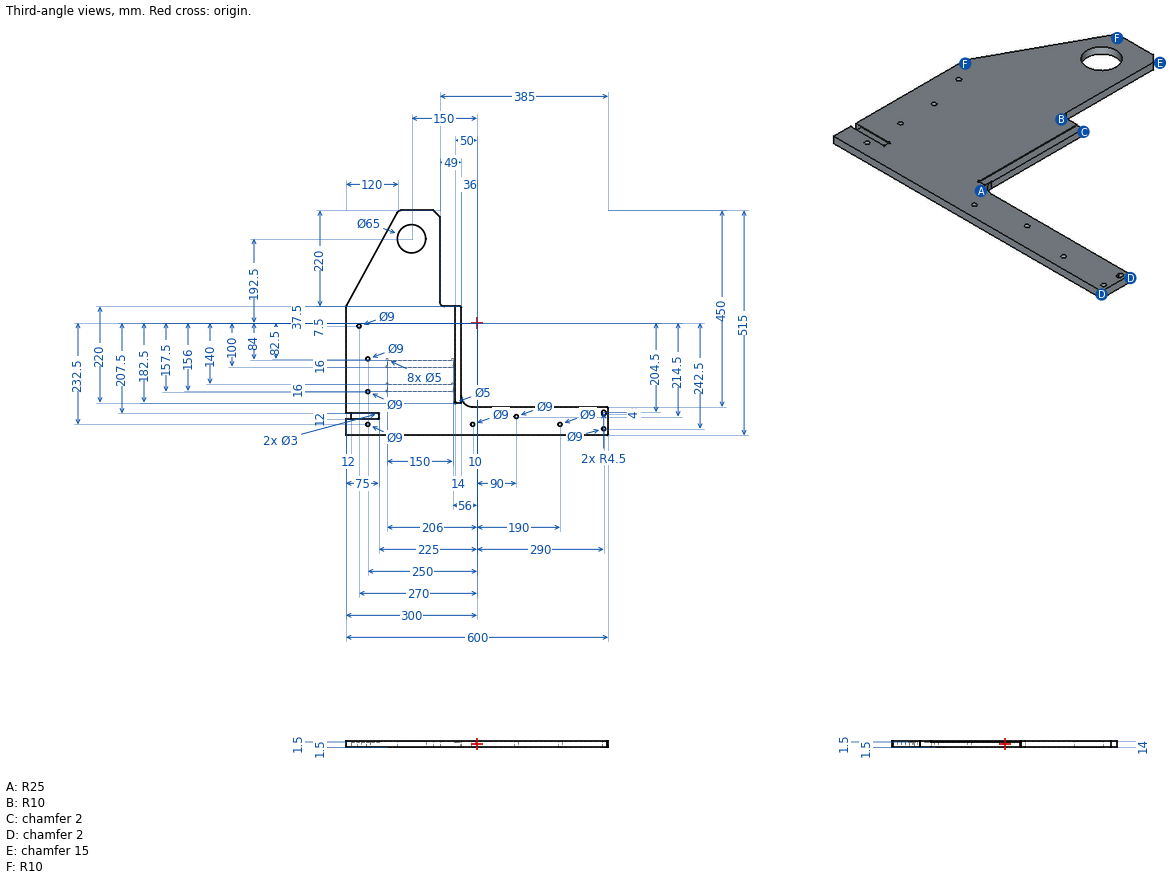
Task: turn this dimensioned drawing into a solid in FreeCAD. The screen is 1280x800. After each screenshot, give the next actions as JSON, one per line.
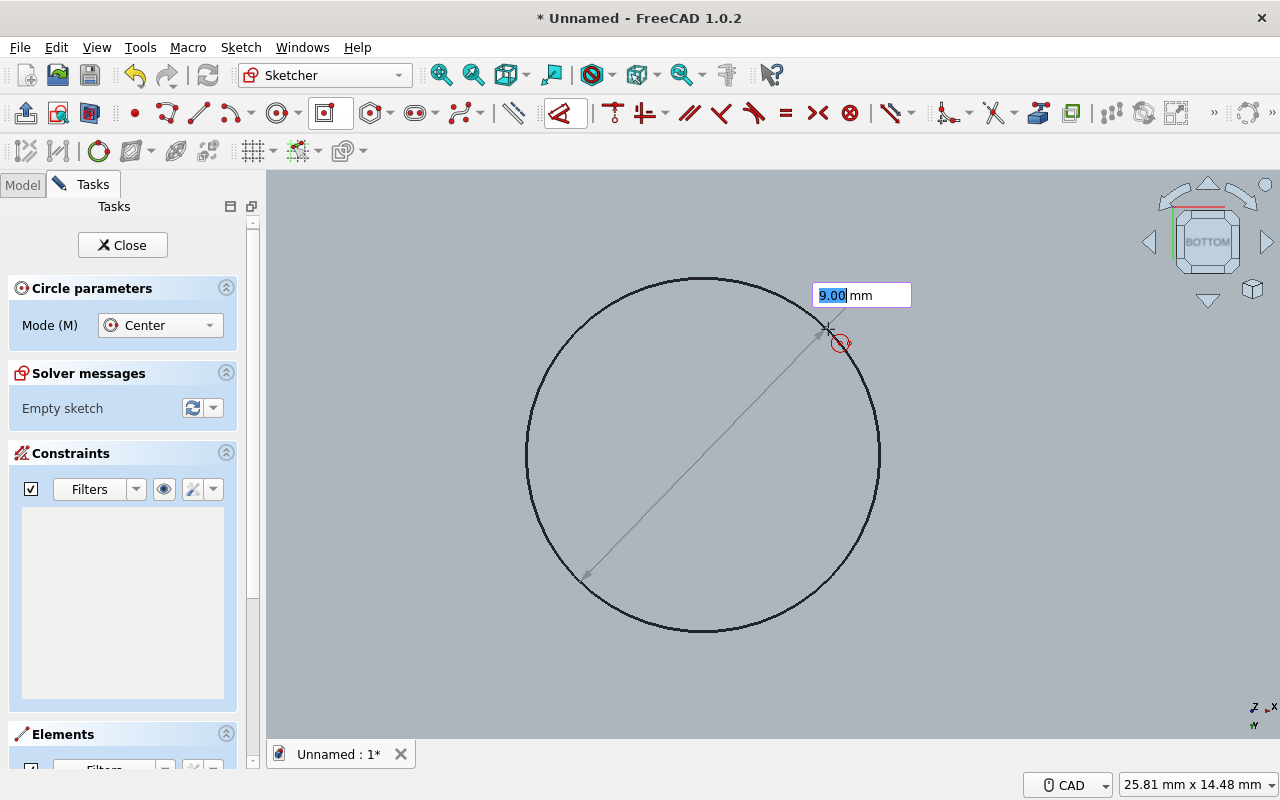
{"action": "type", "text": "9"}
{"action": "key", "text": "Return"}
{"action": "key", "text": "Escape"}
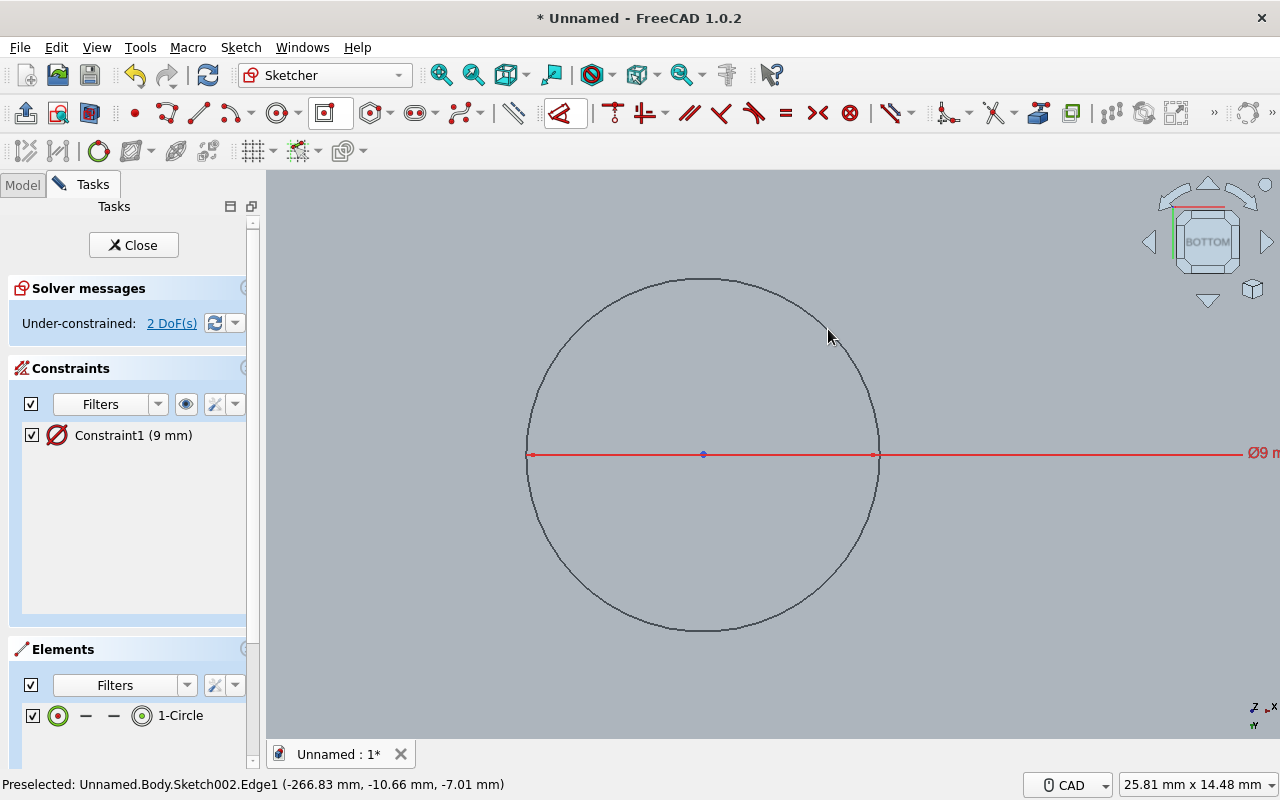
{"action": "left_click", "coordinate": [703, 455]}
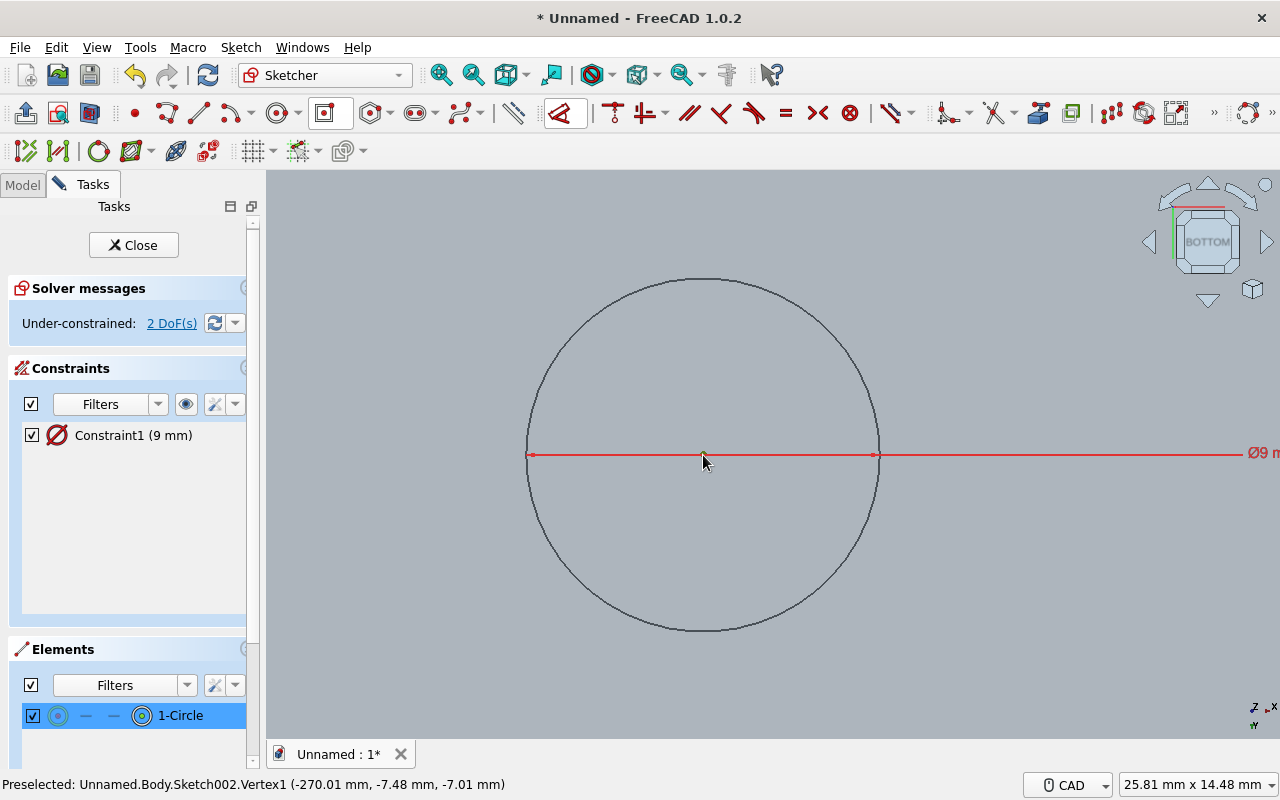
{"action": "left_click", "coordinate": [582, 114]}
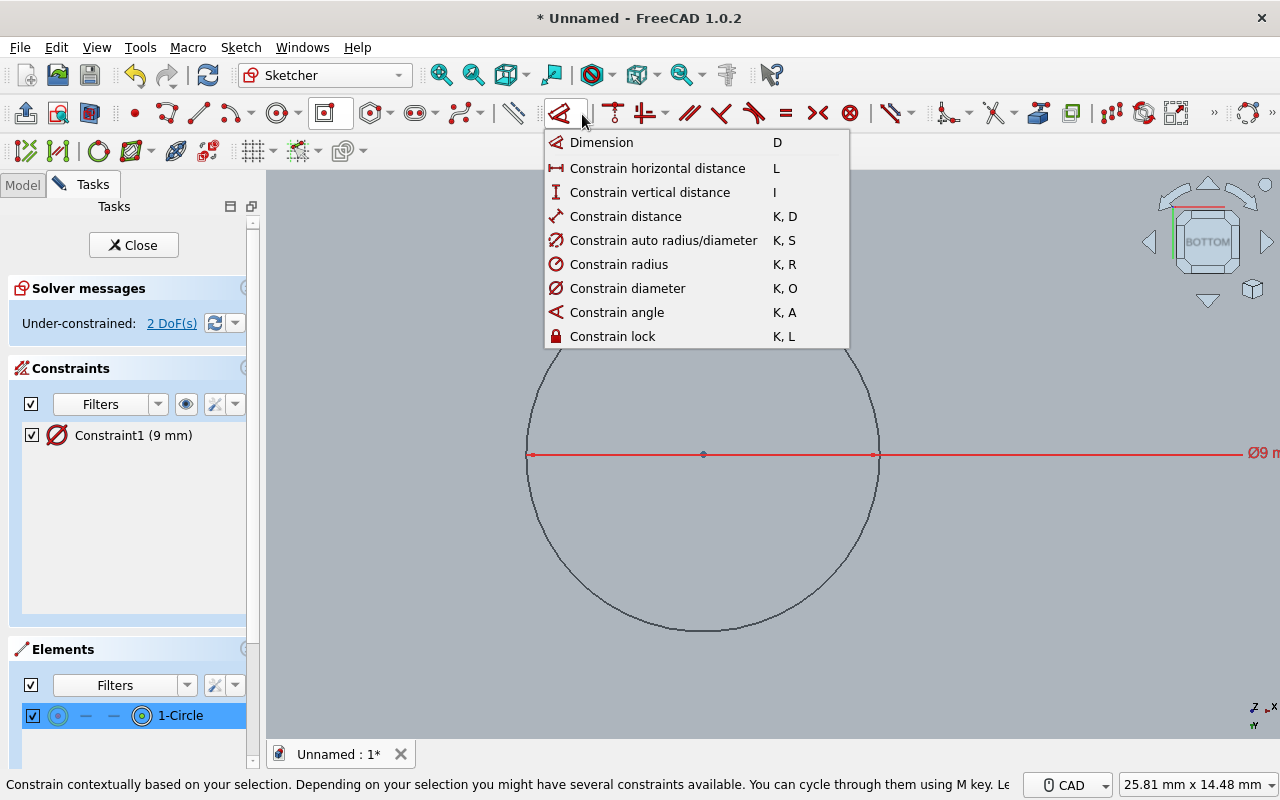
{"action": "left_click", "coordinate": [697, 168]}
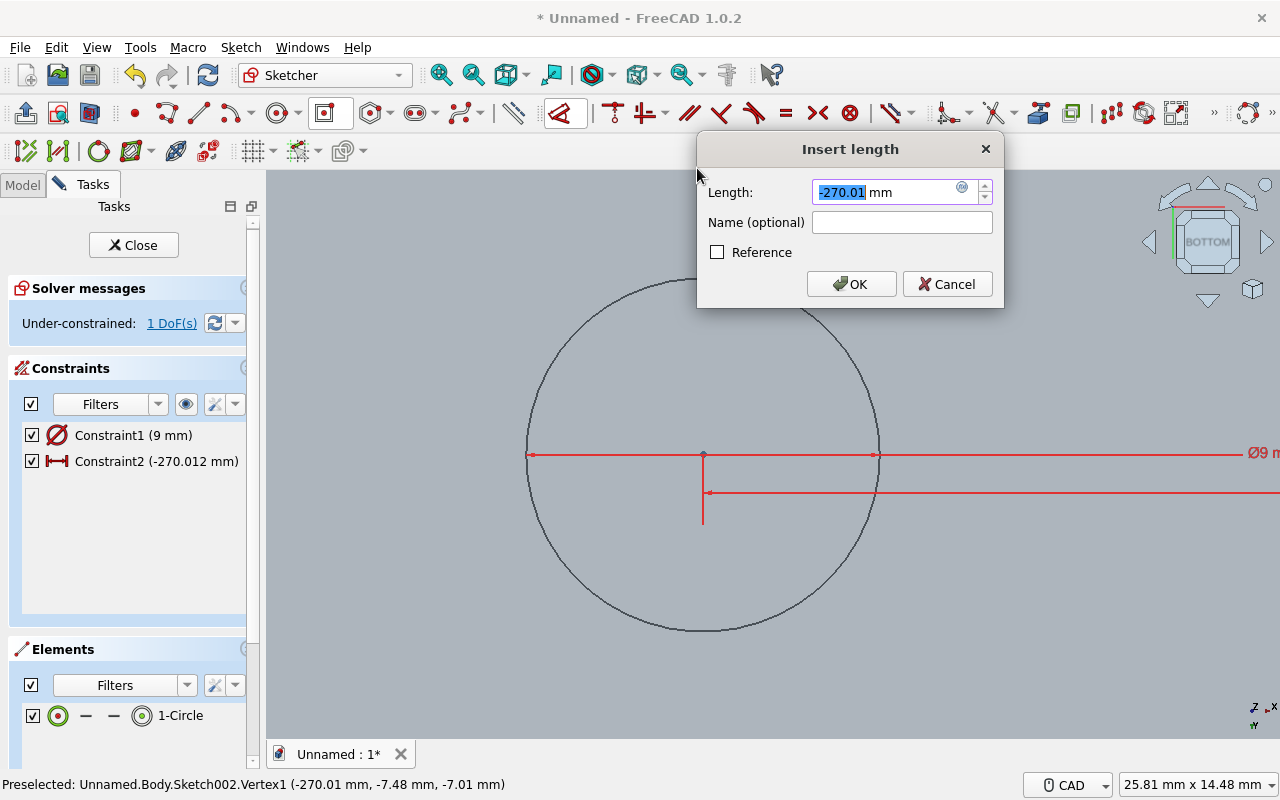
{"action": "type", "text": "-270"}
{"action": "key", "text": "Return"}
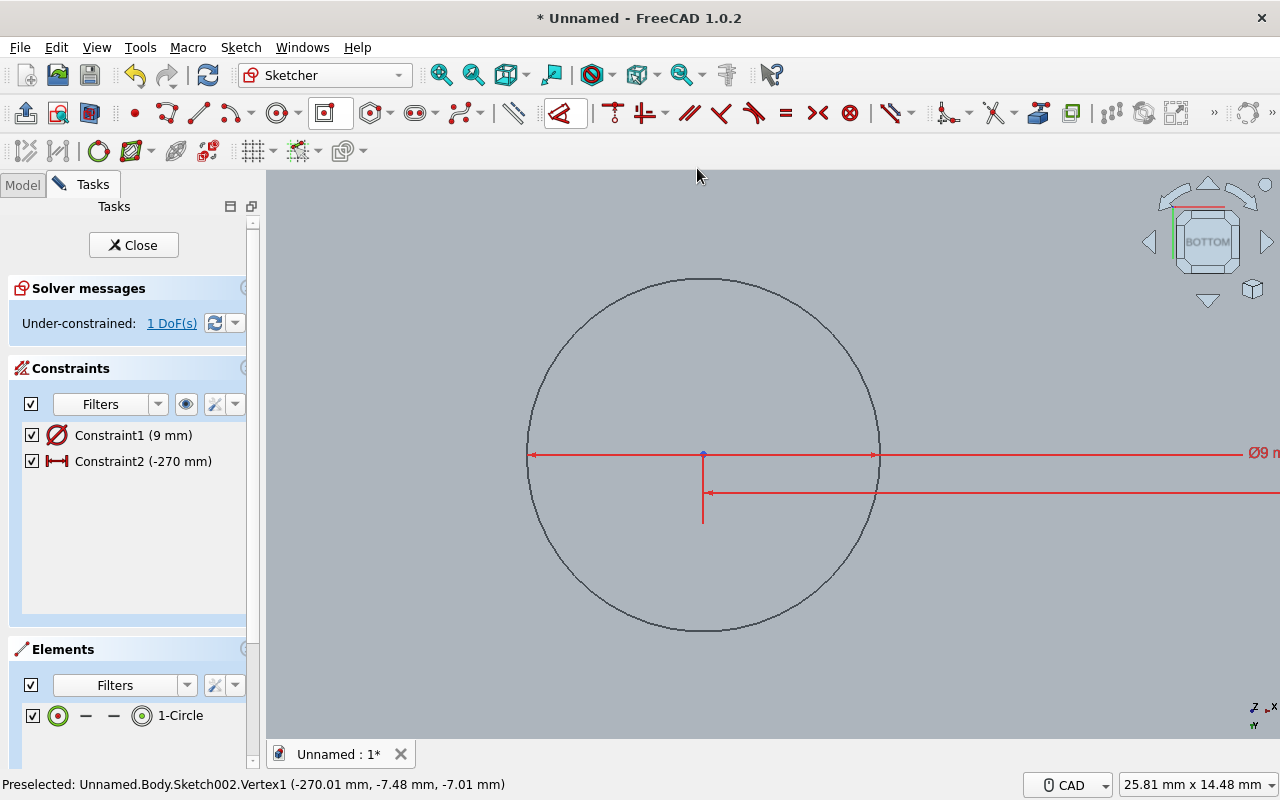
{"action": "left_click", "coordinate": [703, 455]}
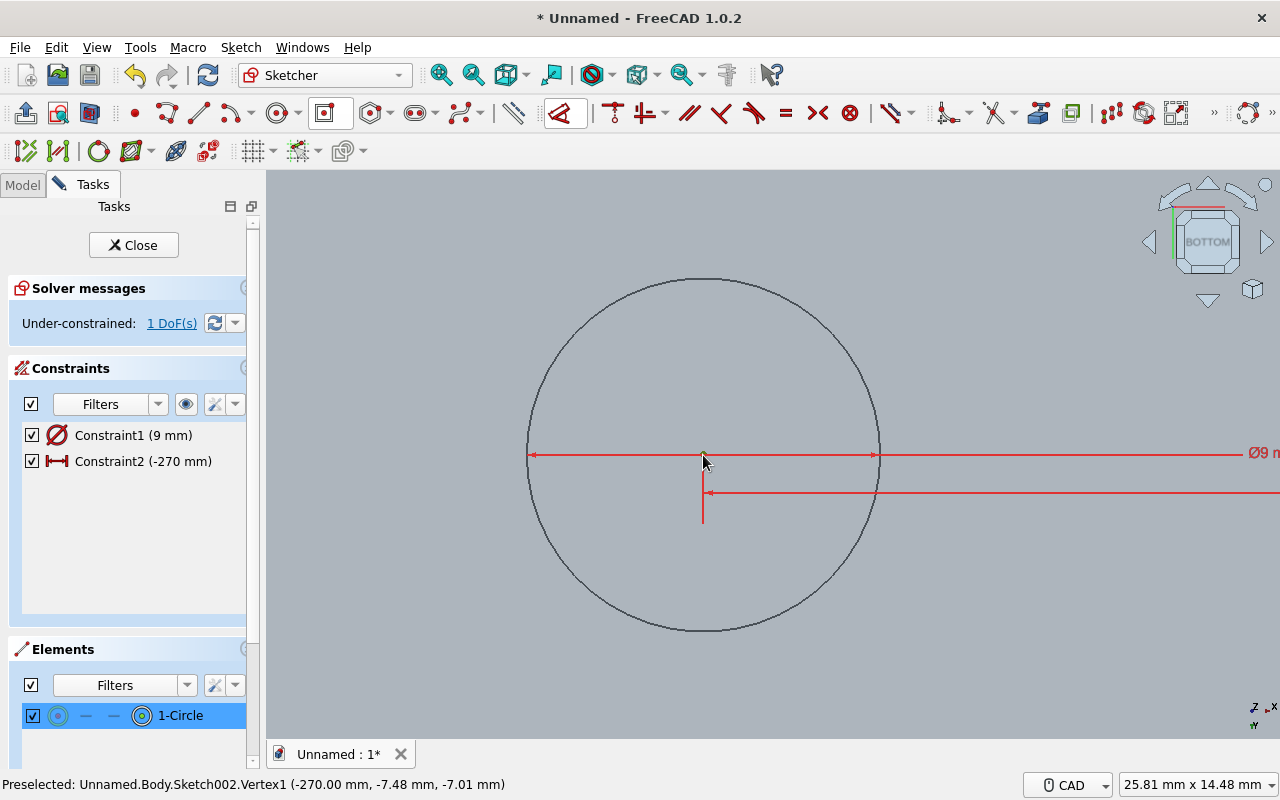
{"action": "key", "text": "i"}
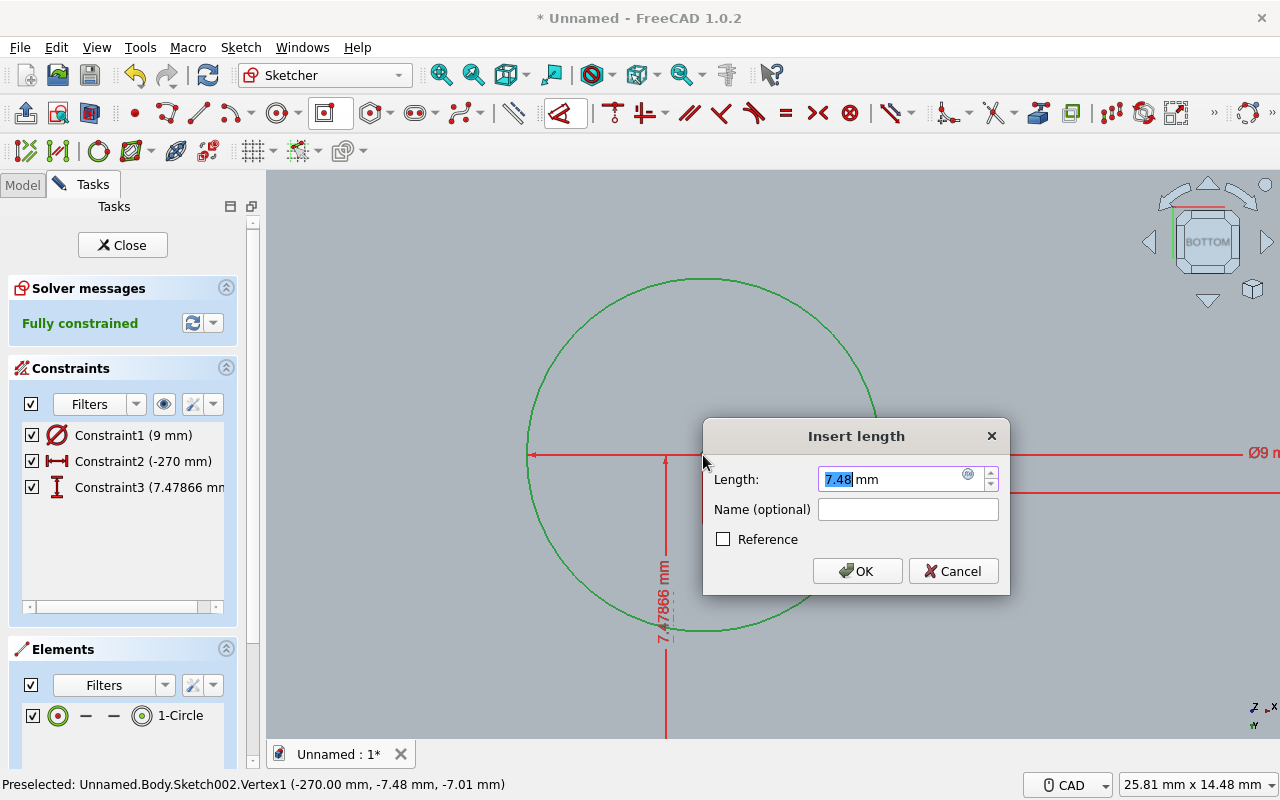
{"action": "type", "text": "7.5"}
{"action": "key", "text": "Return"}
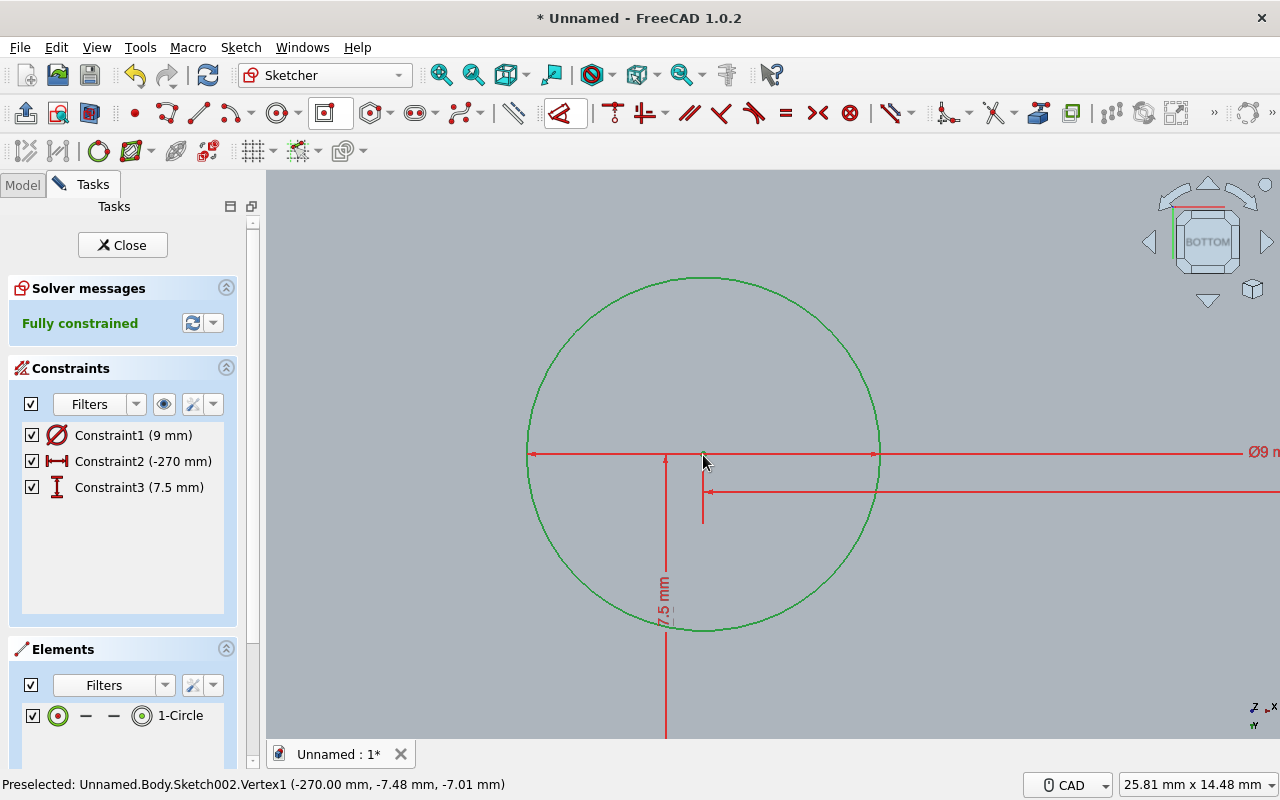
{"action": "left_click", "coordinate": [123, 245]}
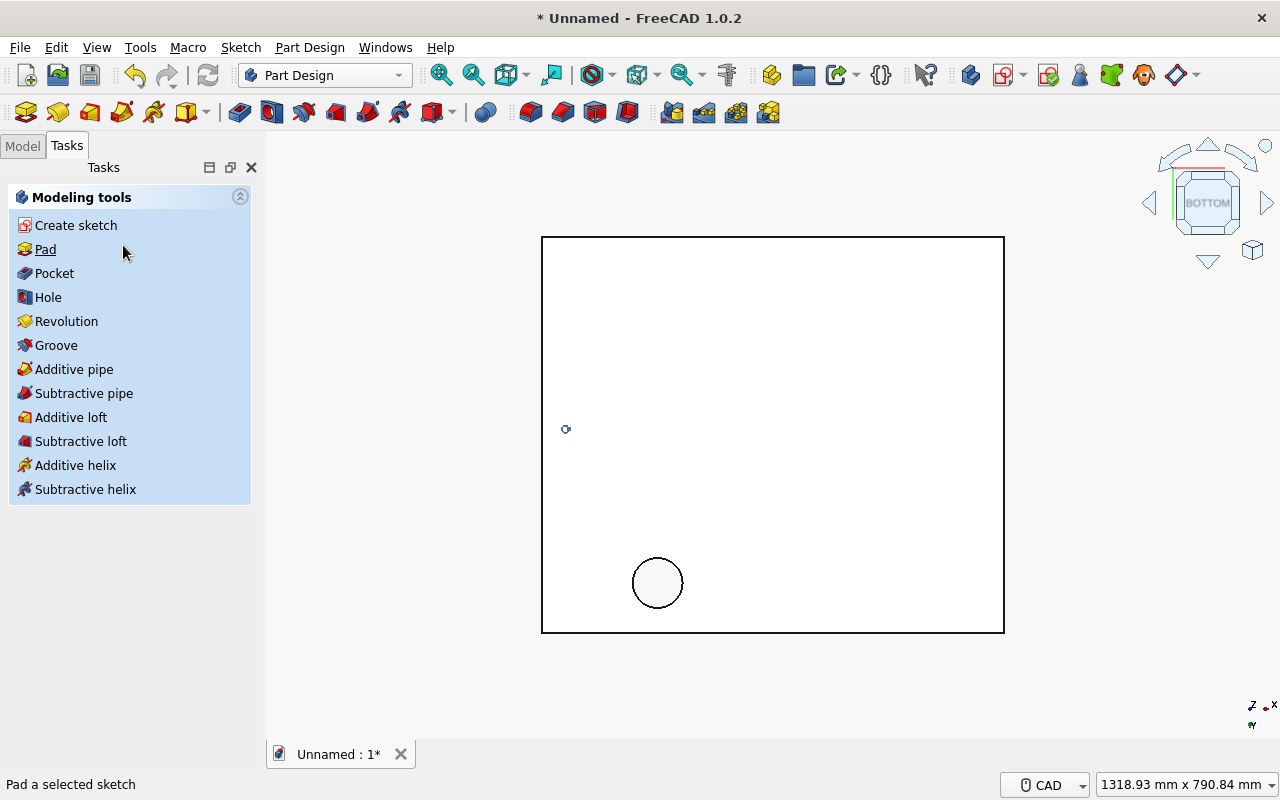
{"action": "left_click", "coordinate": [240, 112]}